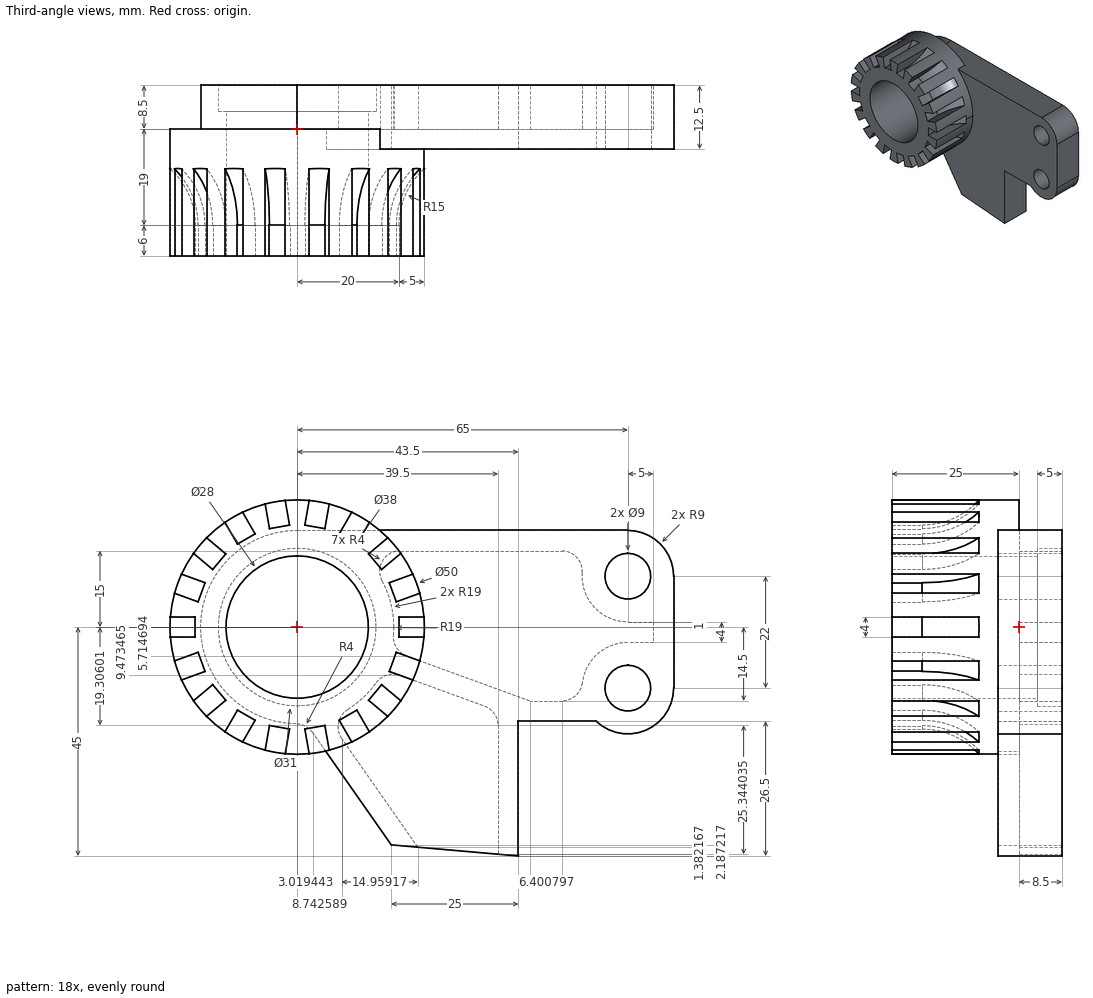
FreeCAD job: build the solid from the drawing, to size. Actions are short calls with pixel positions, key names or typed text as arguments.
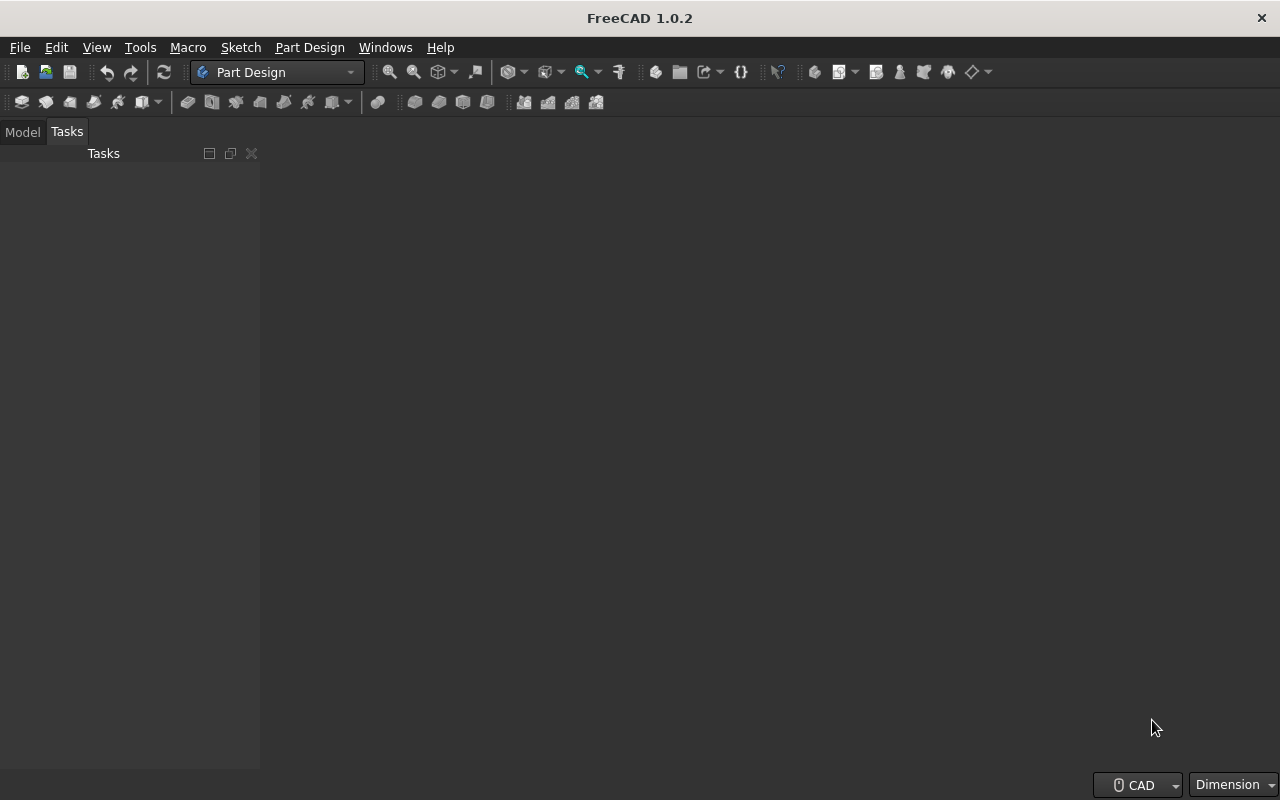
click(22, 72)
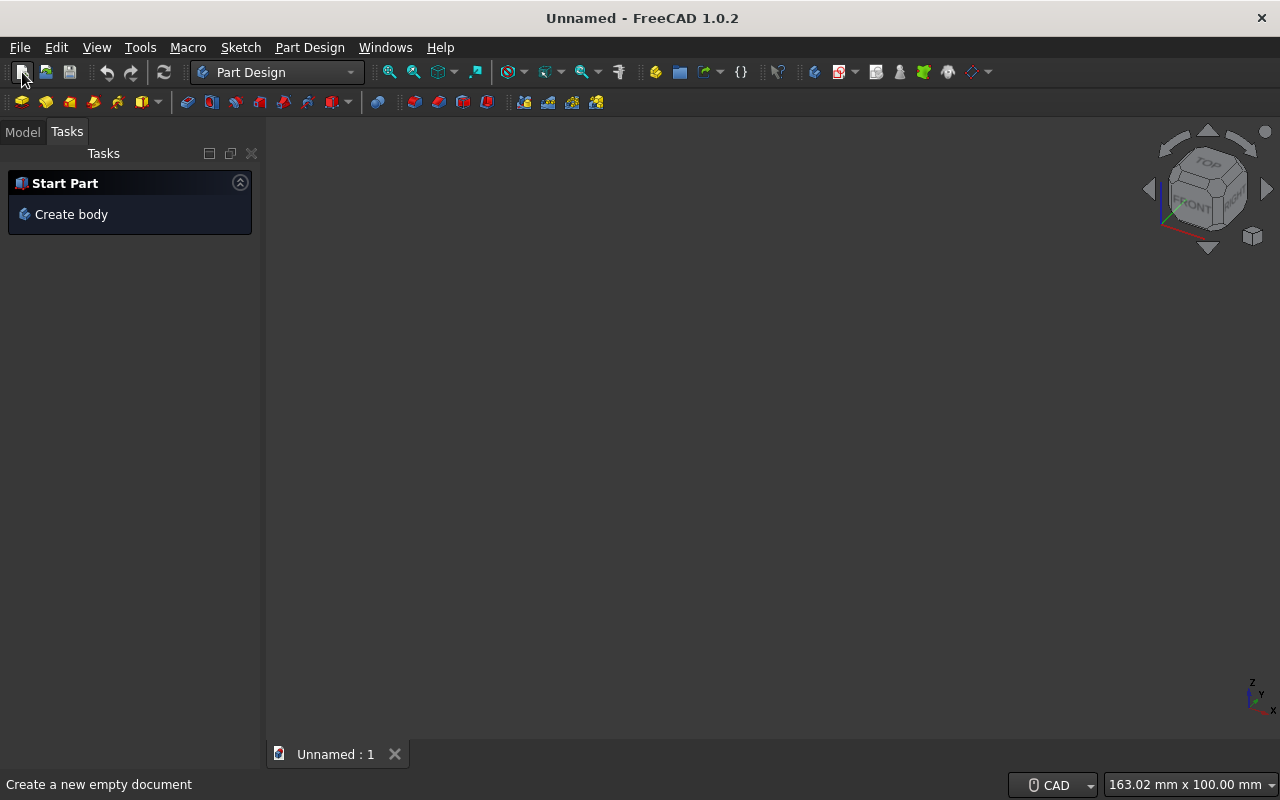
click(840, 72)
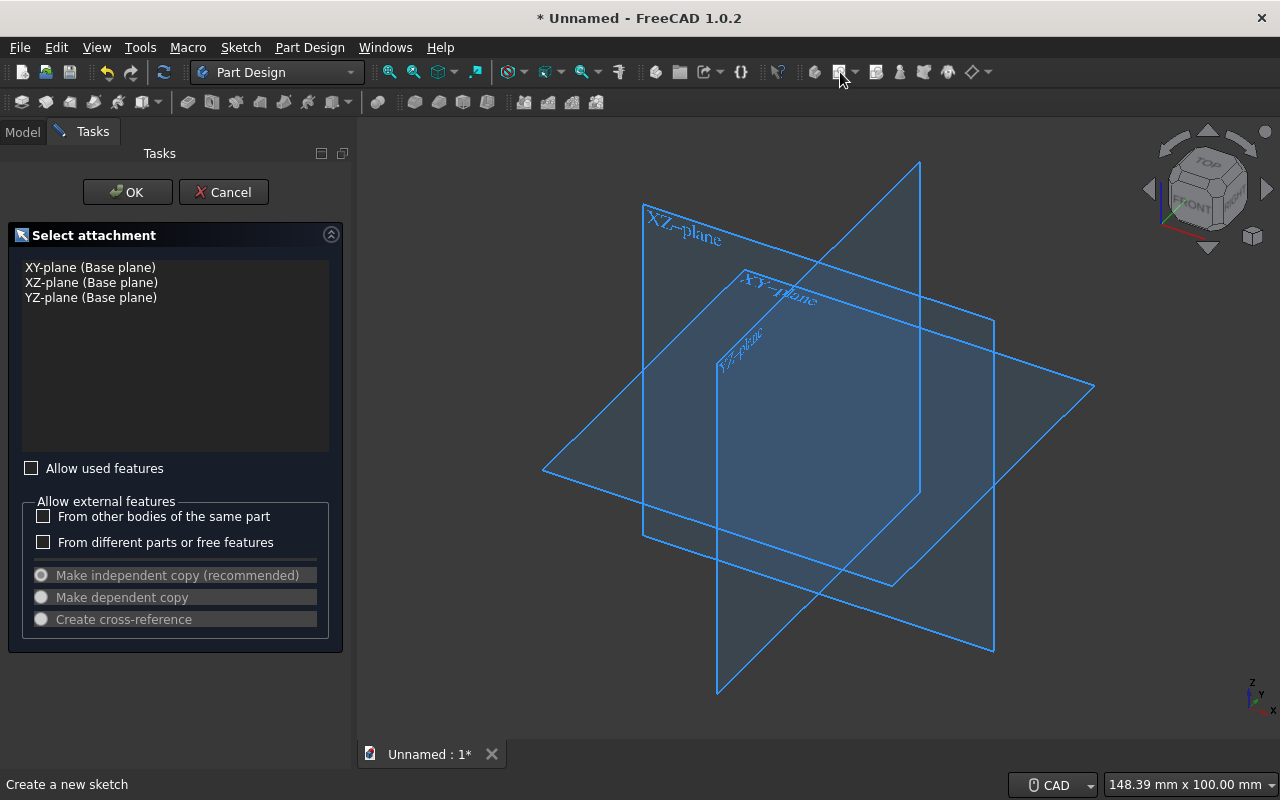
click(82, 282)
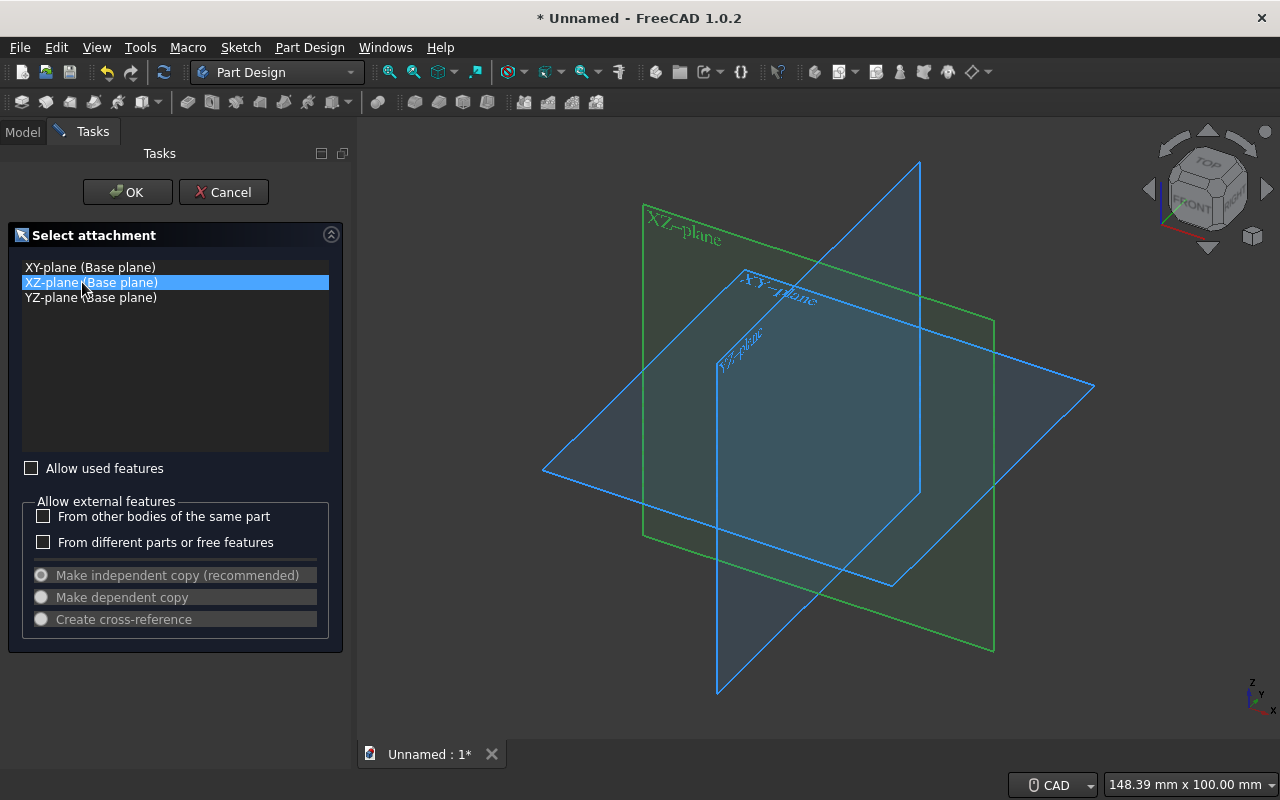
click(128, 192)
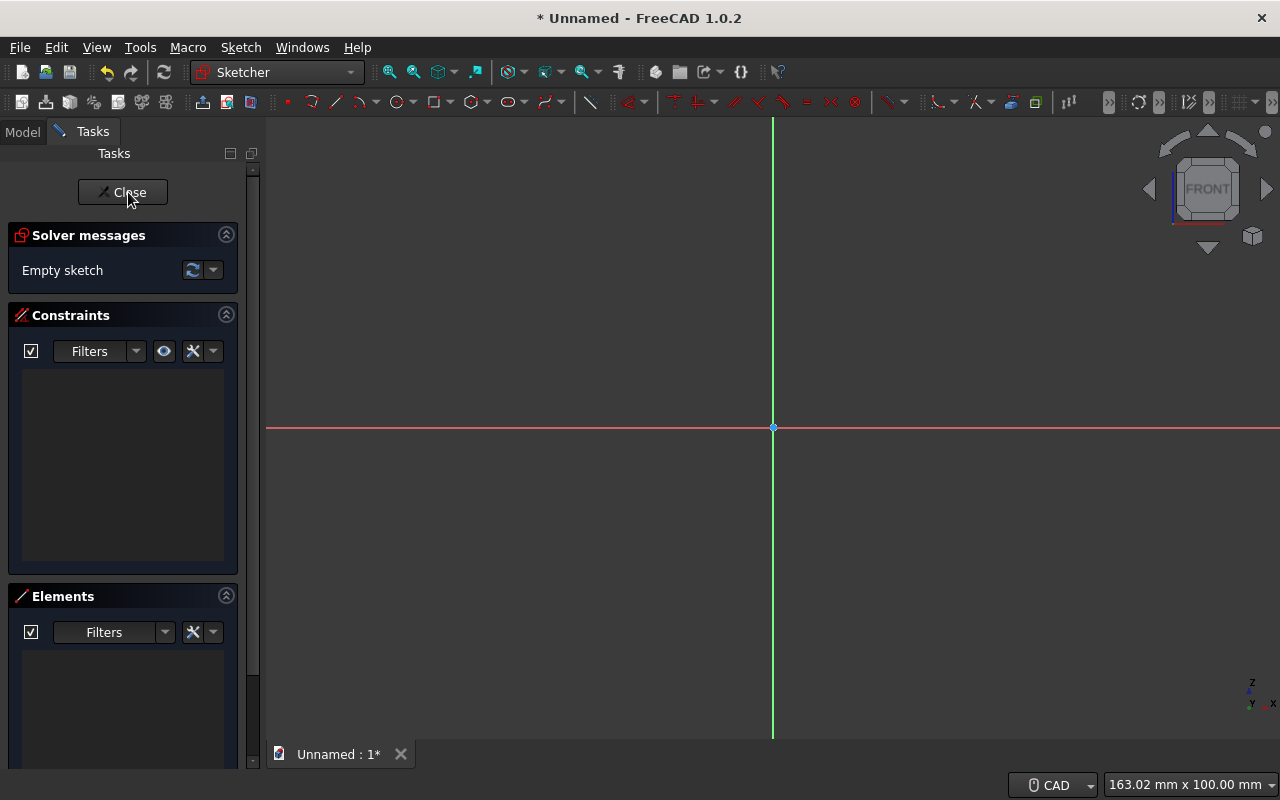
click(398, 102)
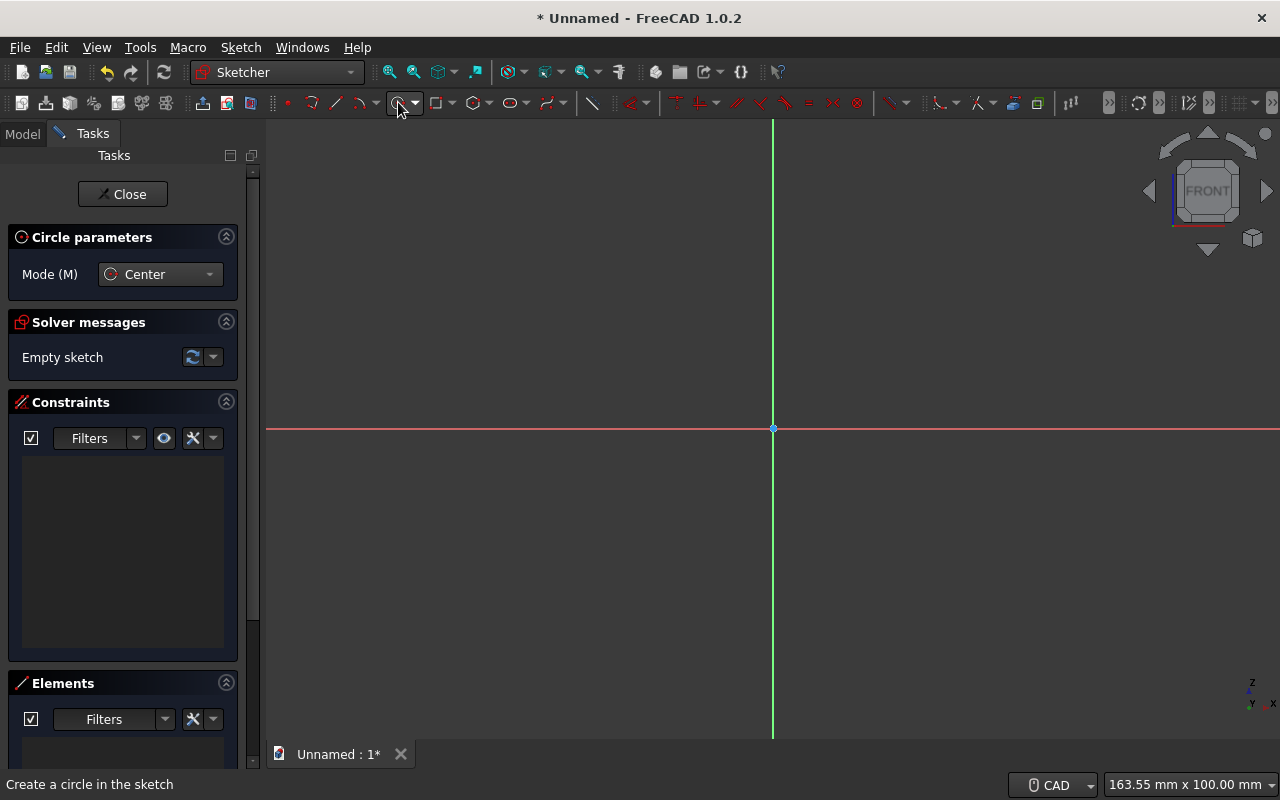
click(773, 429)
move(883, 319)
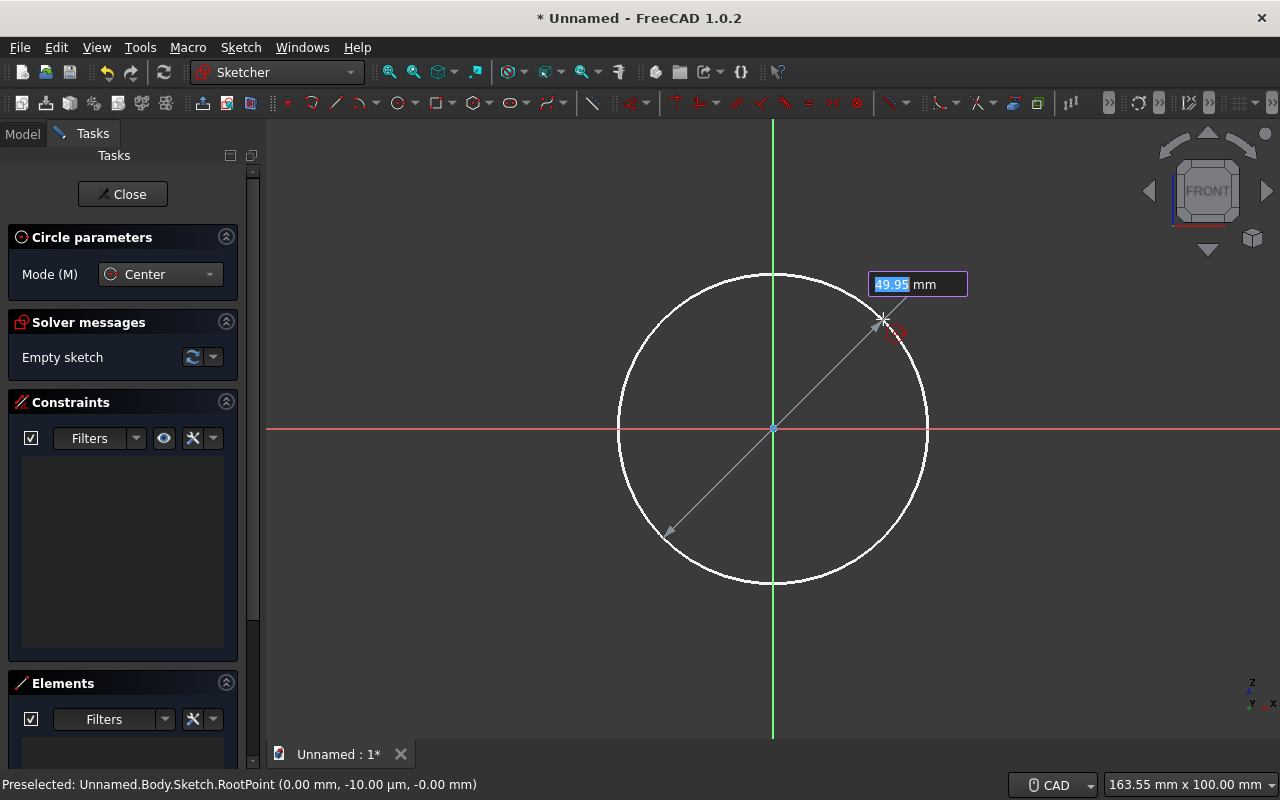
text(50)
key(Return)
key(Escape)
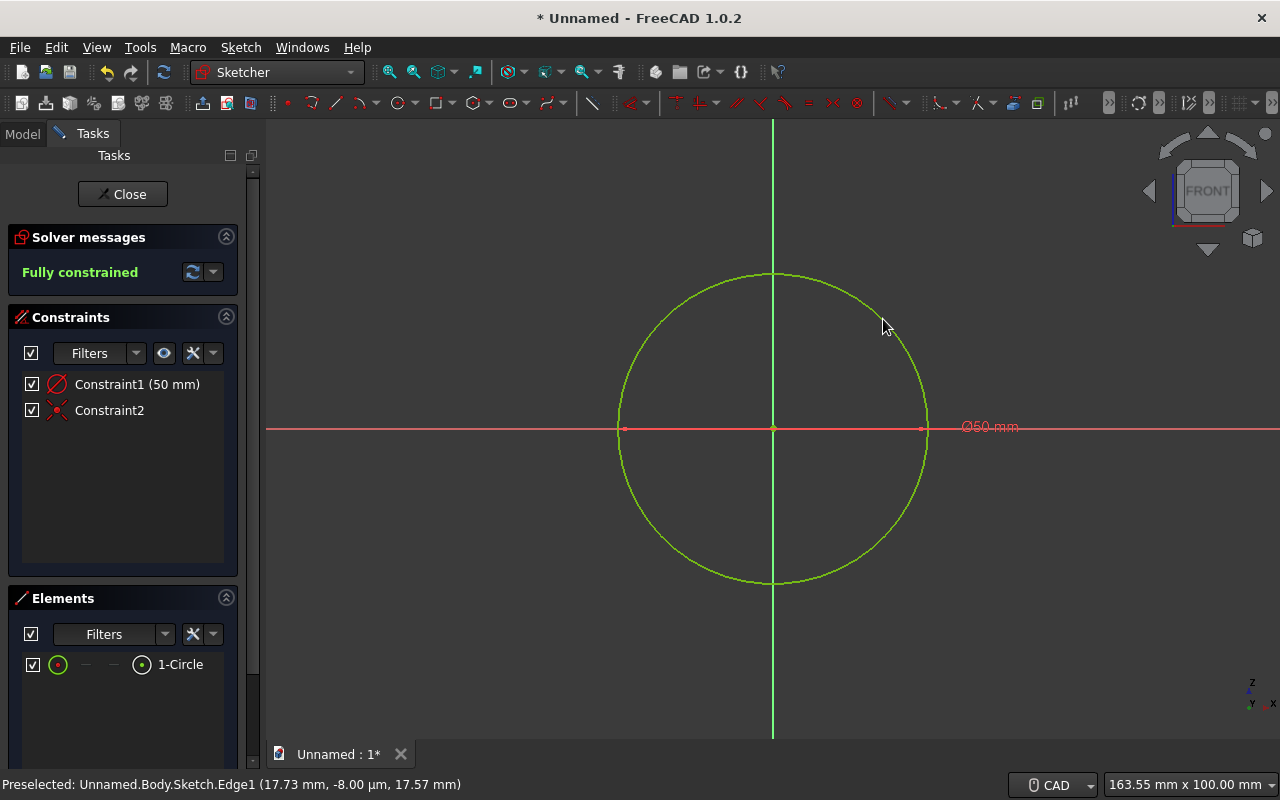
click(123, 194)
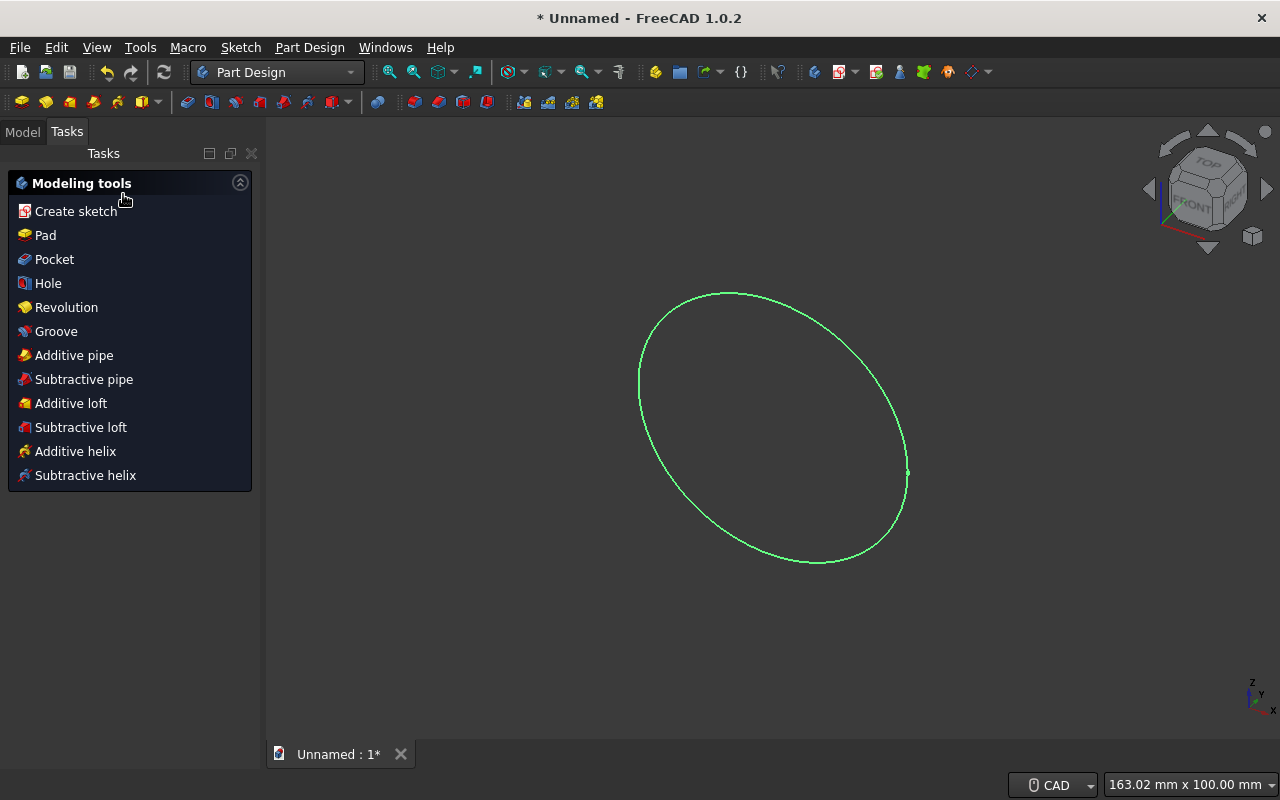
click(22, 102)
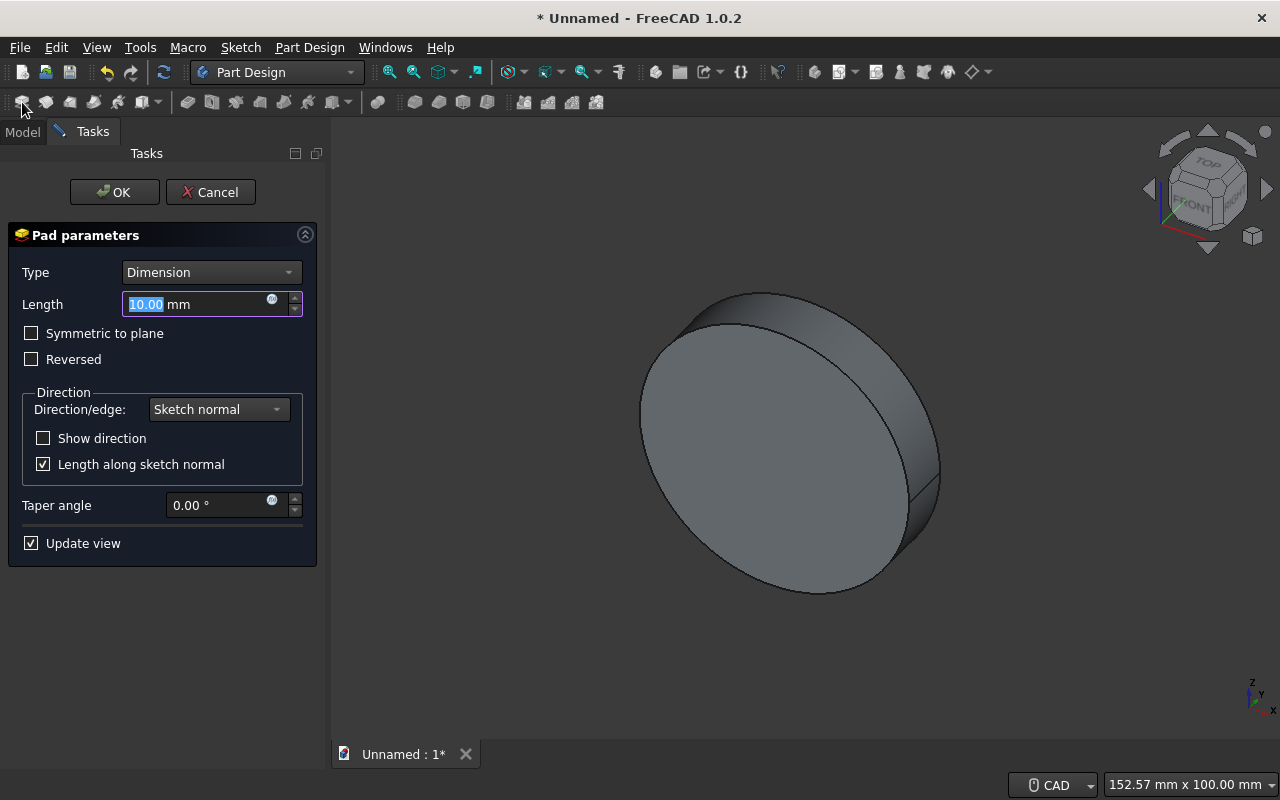
text(25)
key(Tab)